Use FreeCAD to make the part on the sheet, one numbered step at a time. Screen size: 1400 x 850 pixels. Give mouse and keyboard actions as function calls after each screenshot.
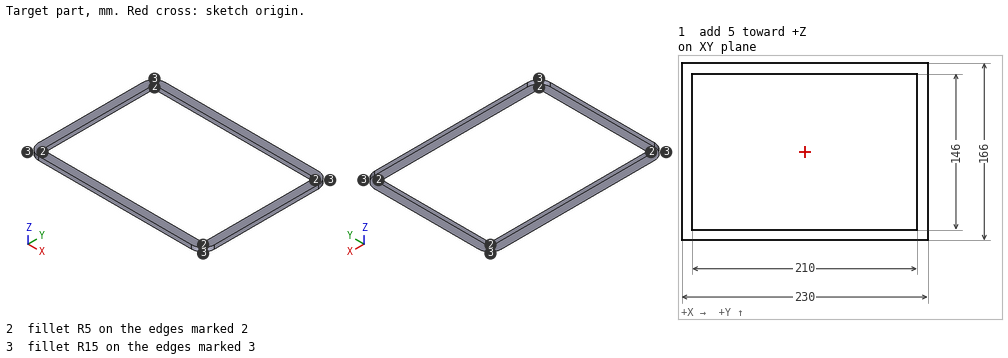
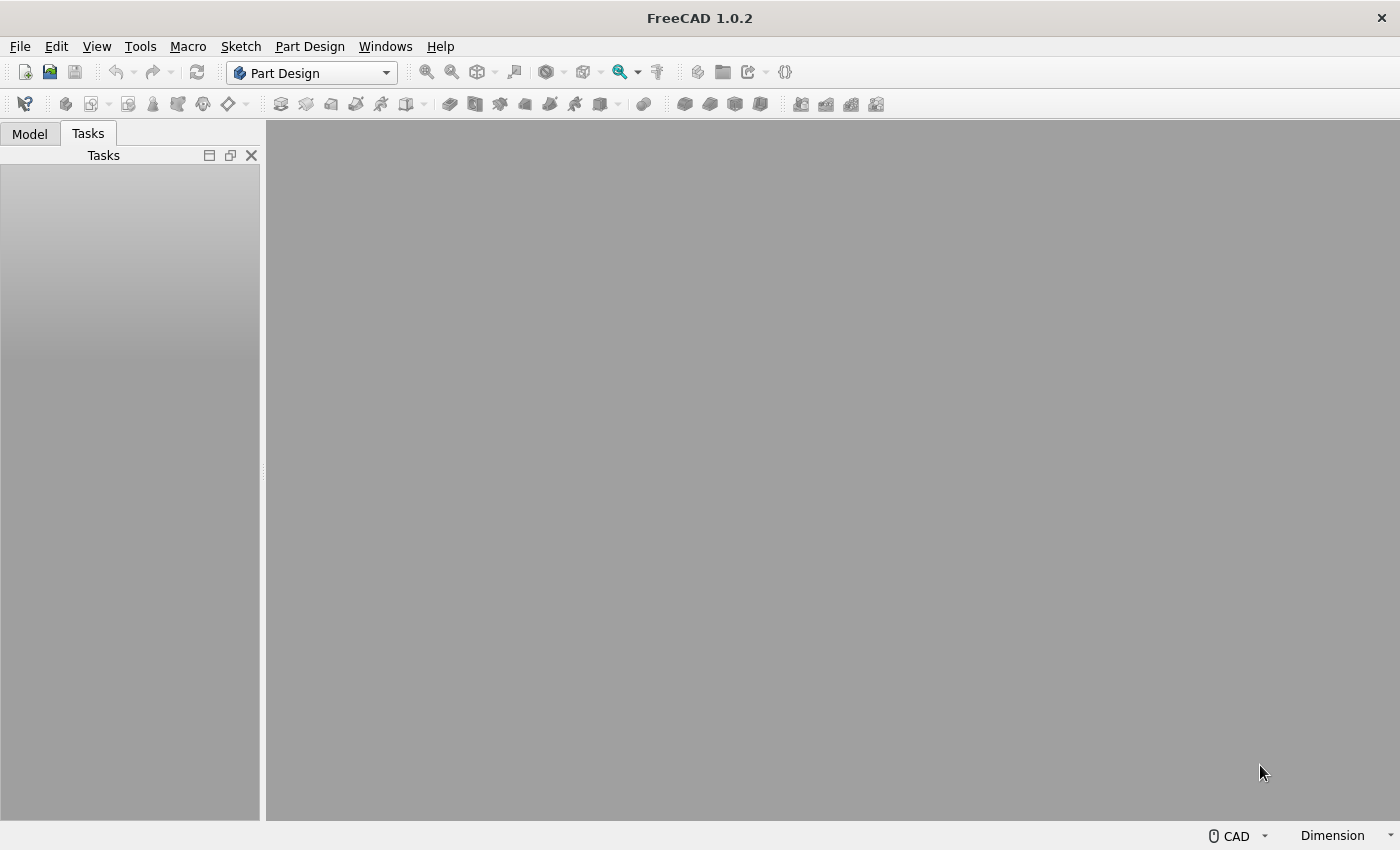
key(ctrl+n)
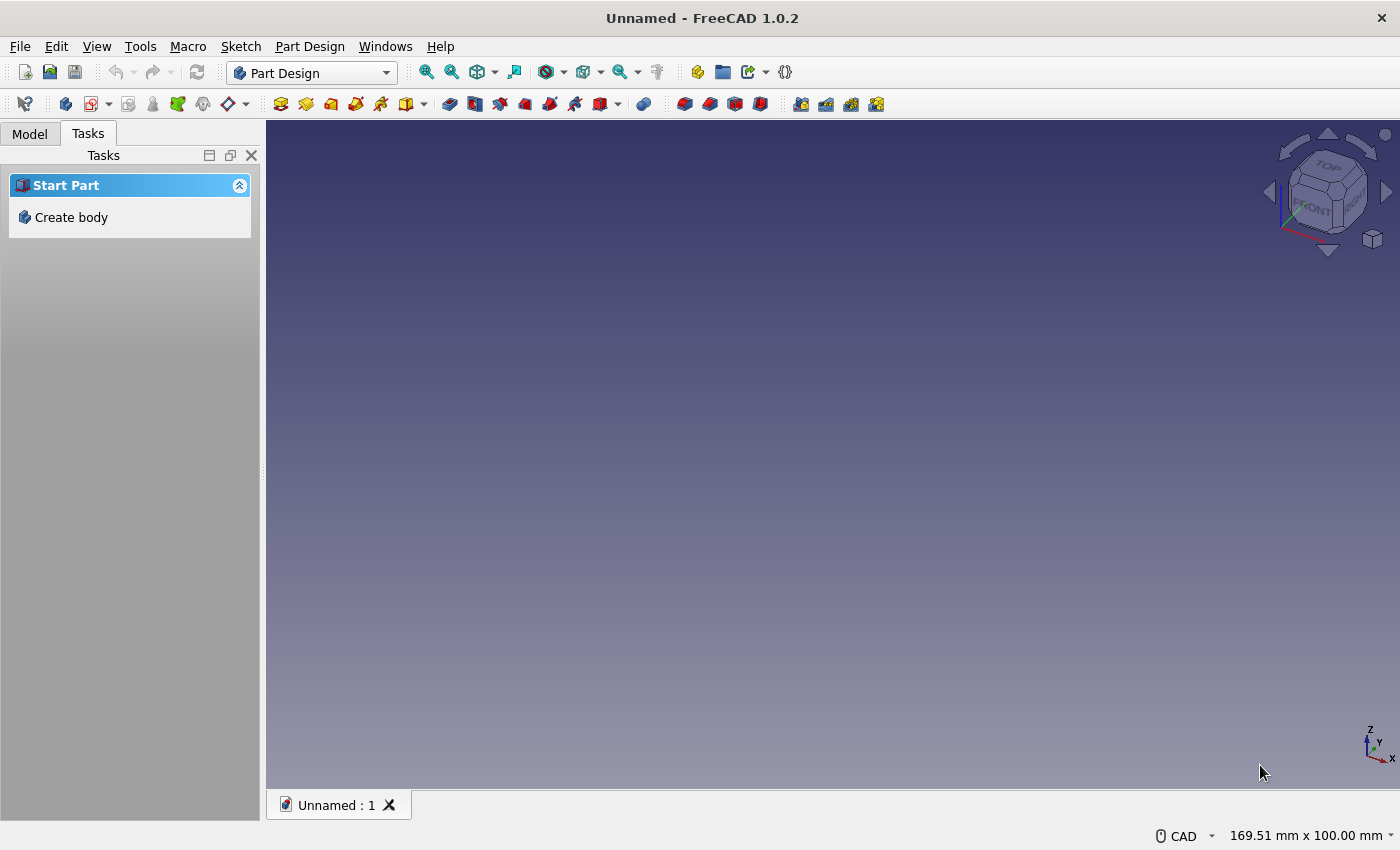
click(90, 104)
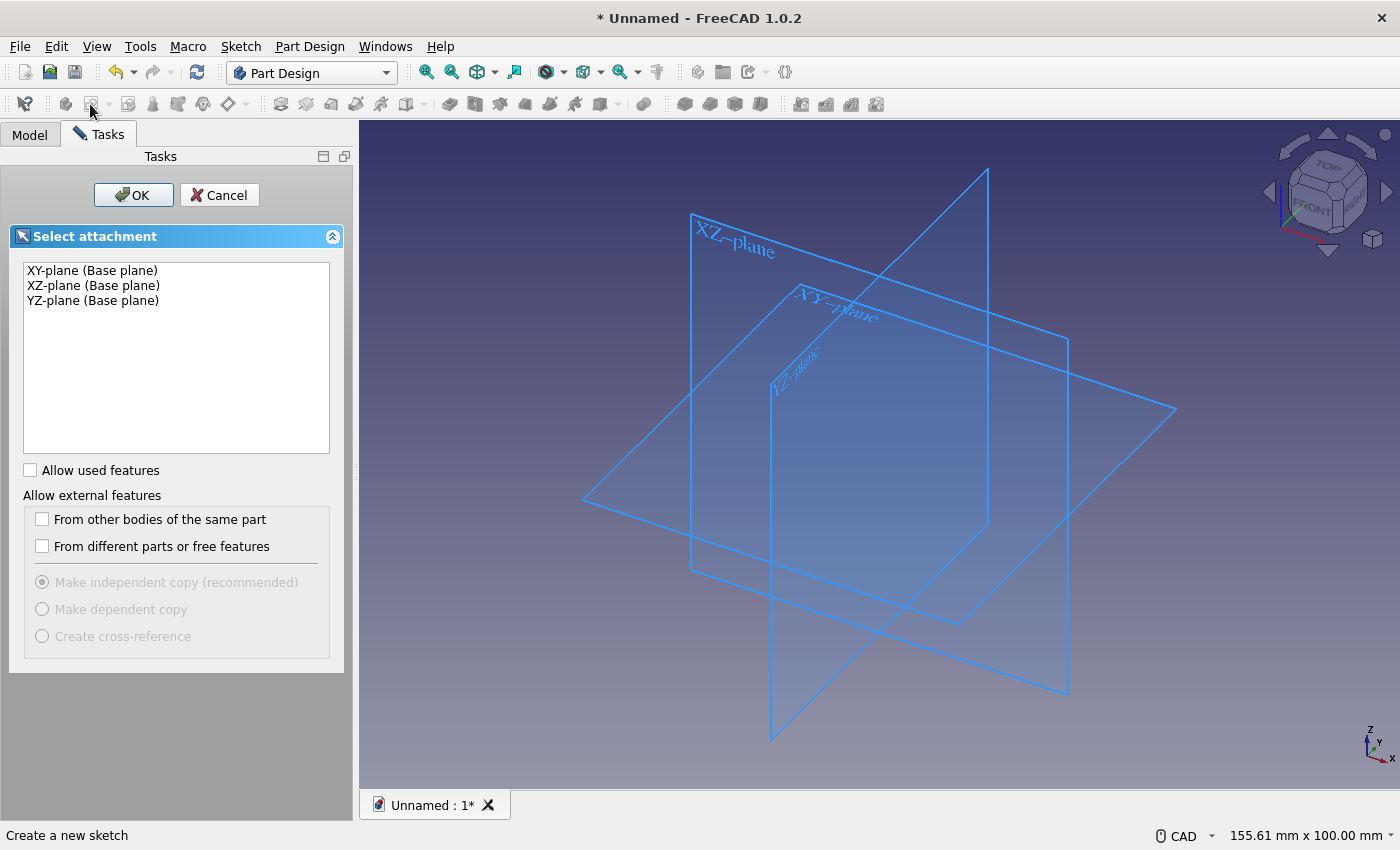
click(84, 270)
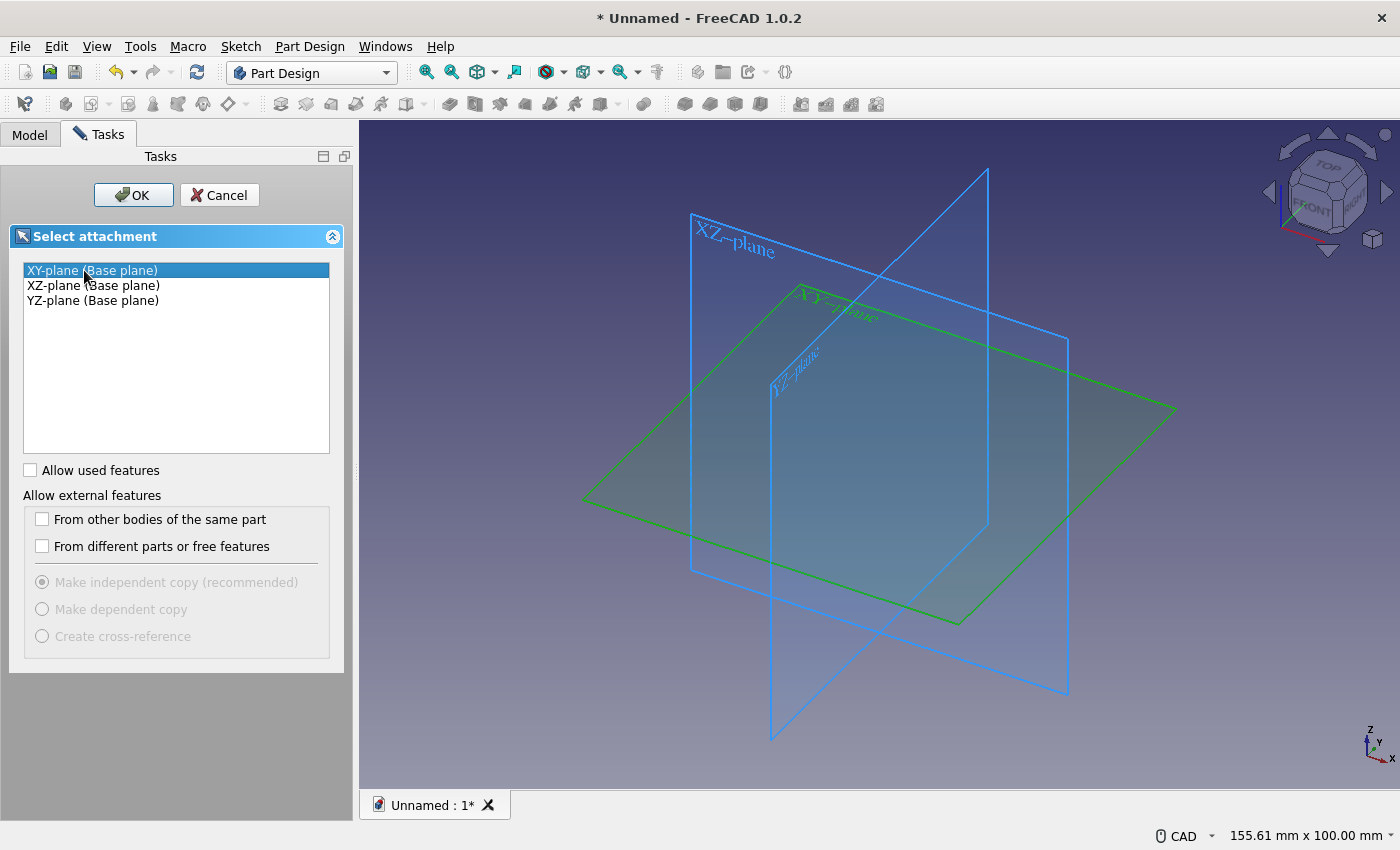
click(134, 195)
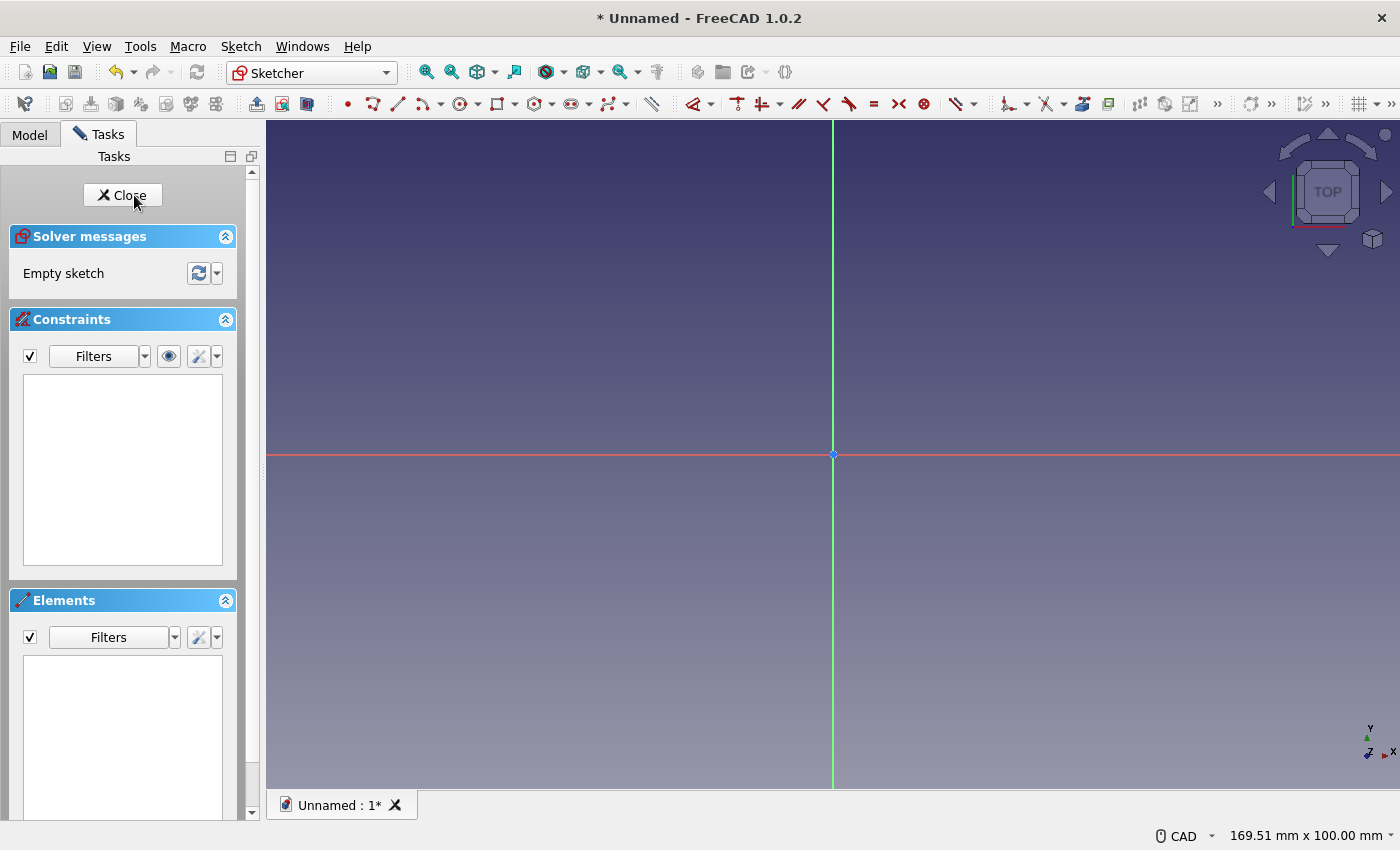
scroll(725, 454, down, 5)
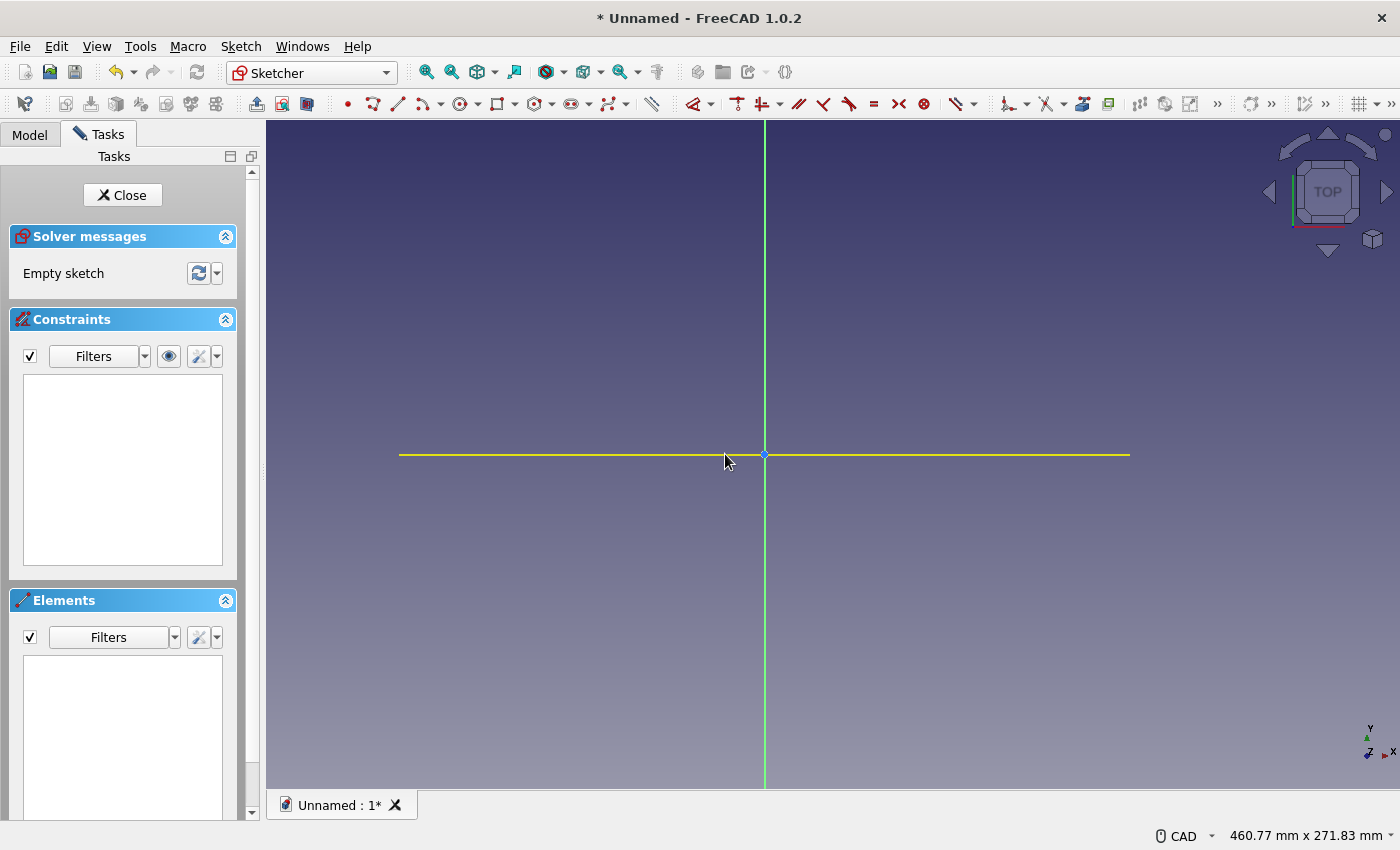
key(g)
key(v)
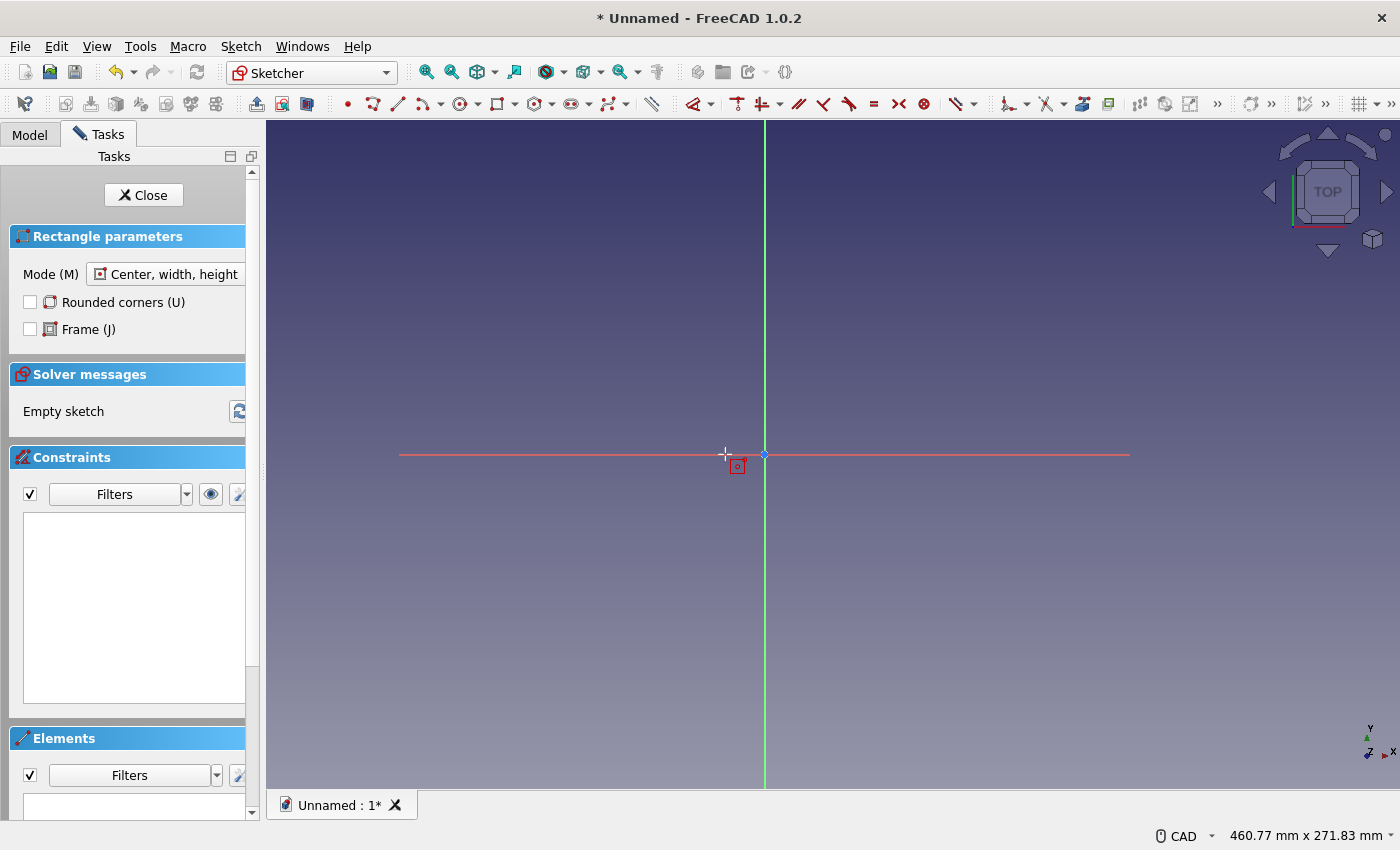
click(765, 454)
click(1048, 250)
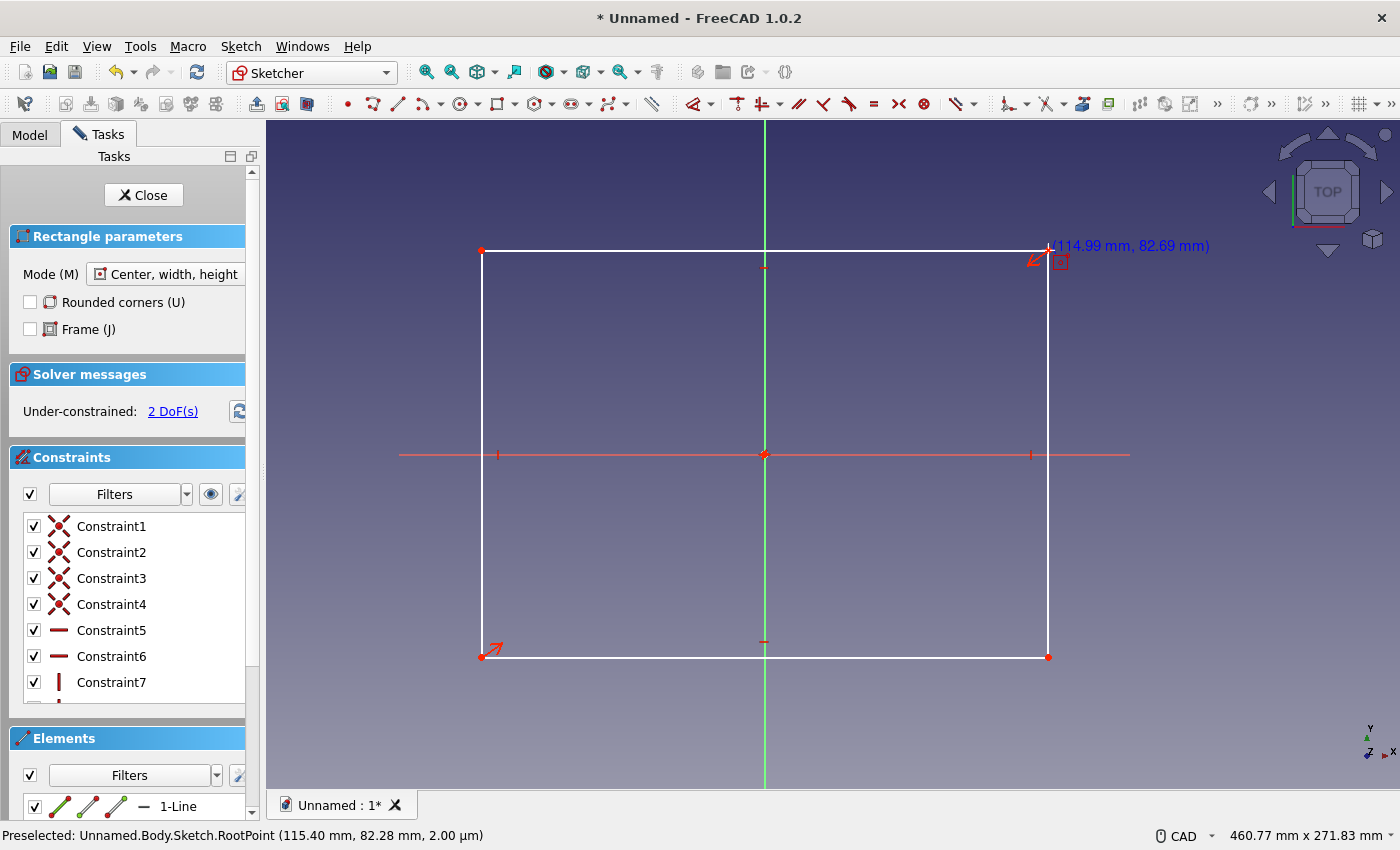
click(765, 454)
click(1023, 275)
key(Escape)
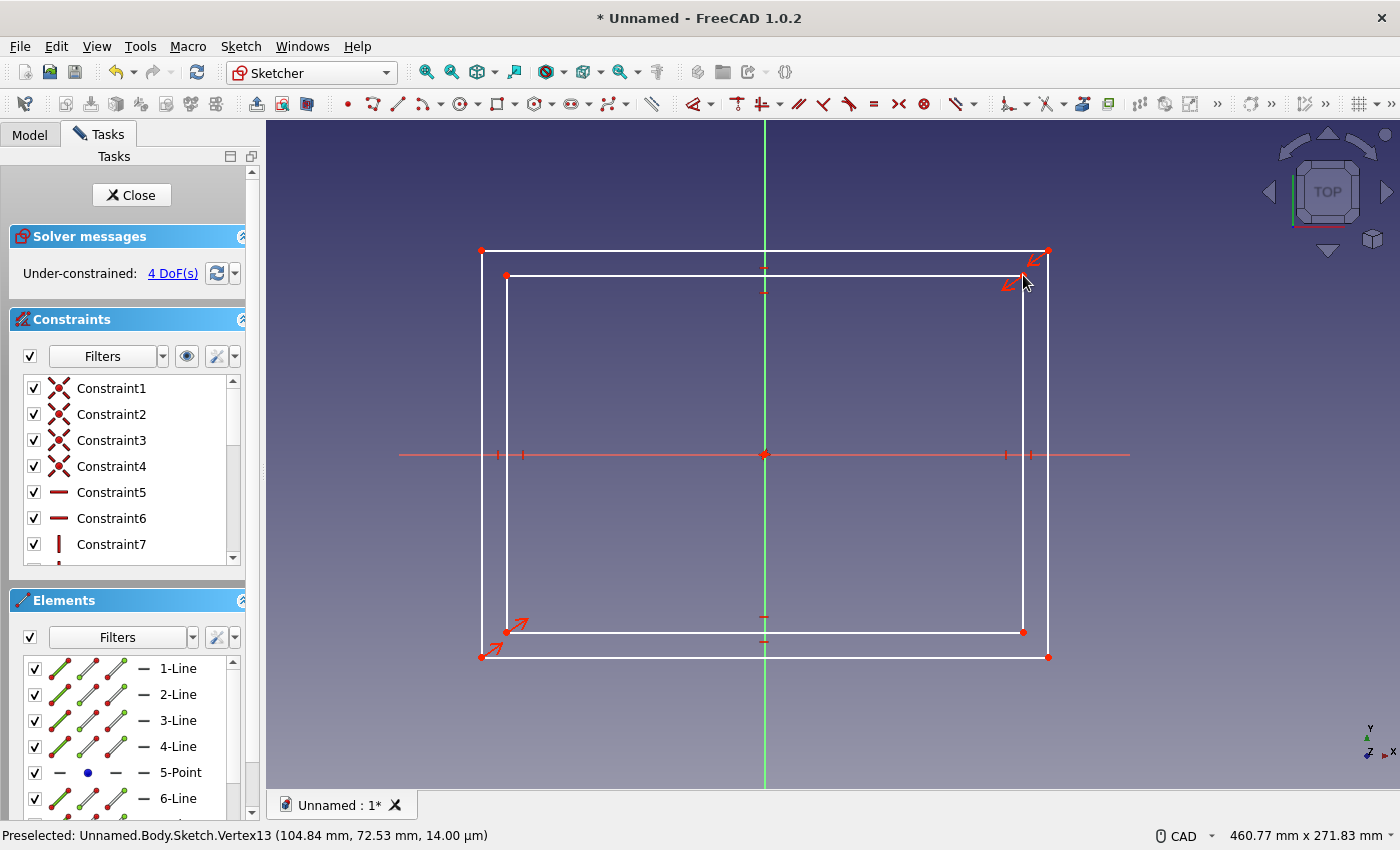
key(d)